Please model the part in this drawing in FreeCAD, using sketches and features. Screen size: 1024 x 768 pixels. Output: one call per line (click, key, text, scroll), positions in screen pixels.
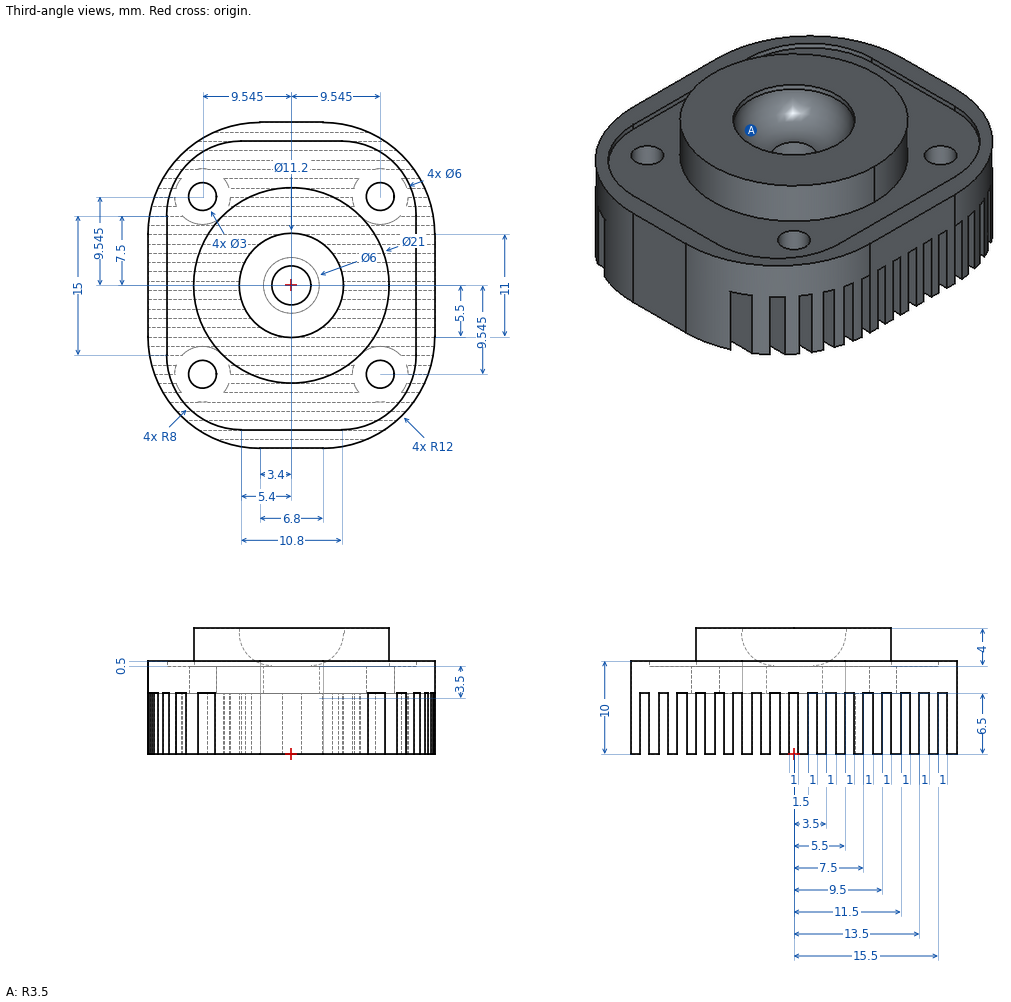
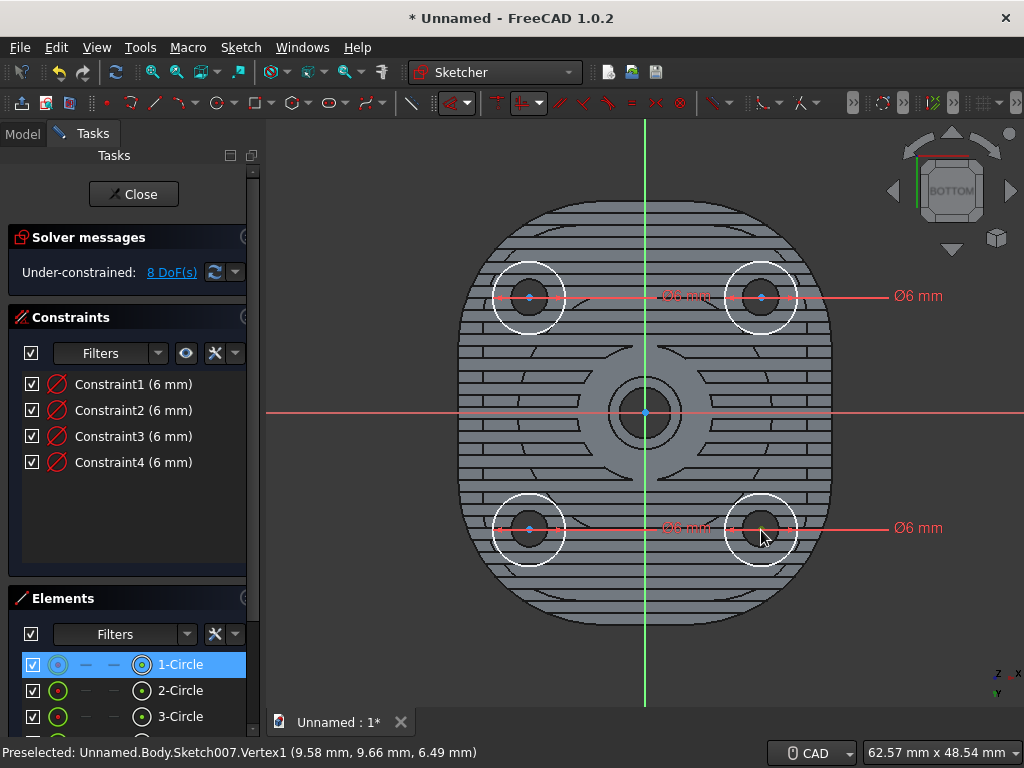
click(529, 530)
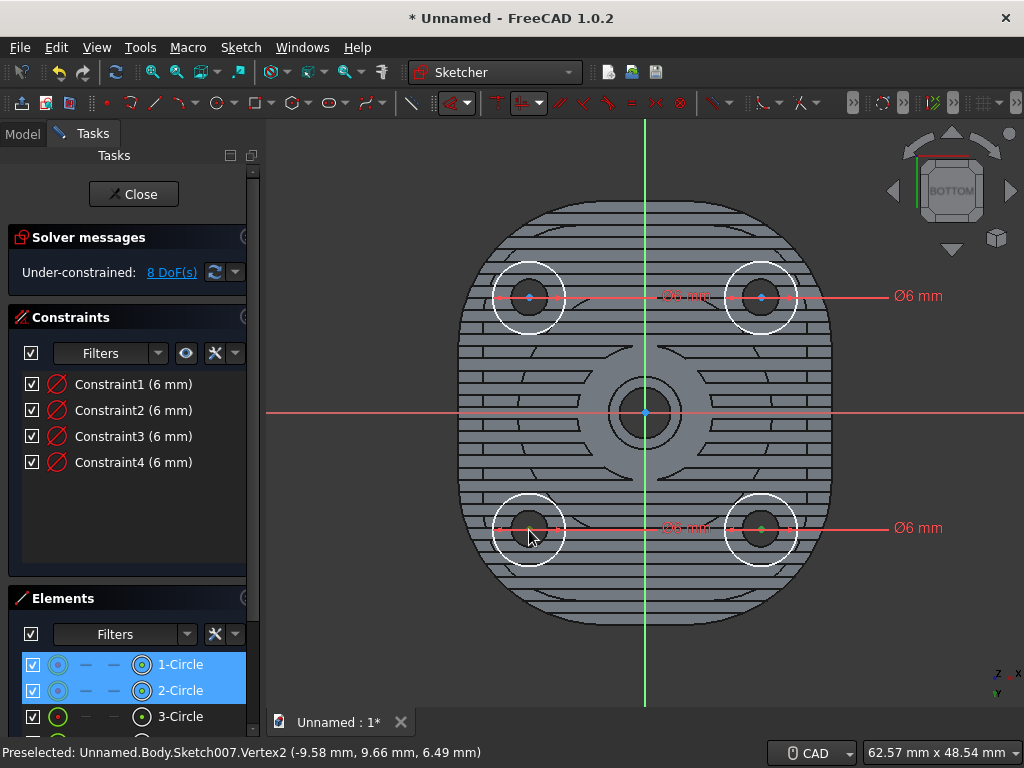
key(h)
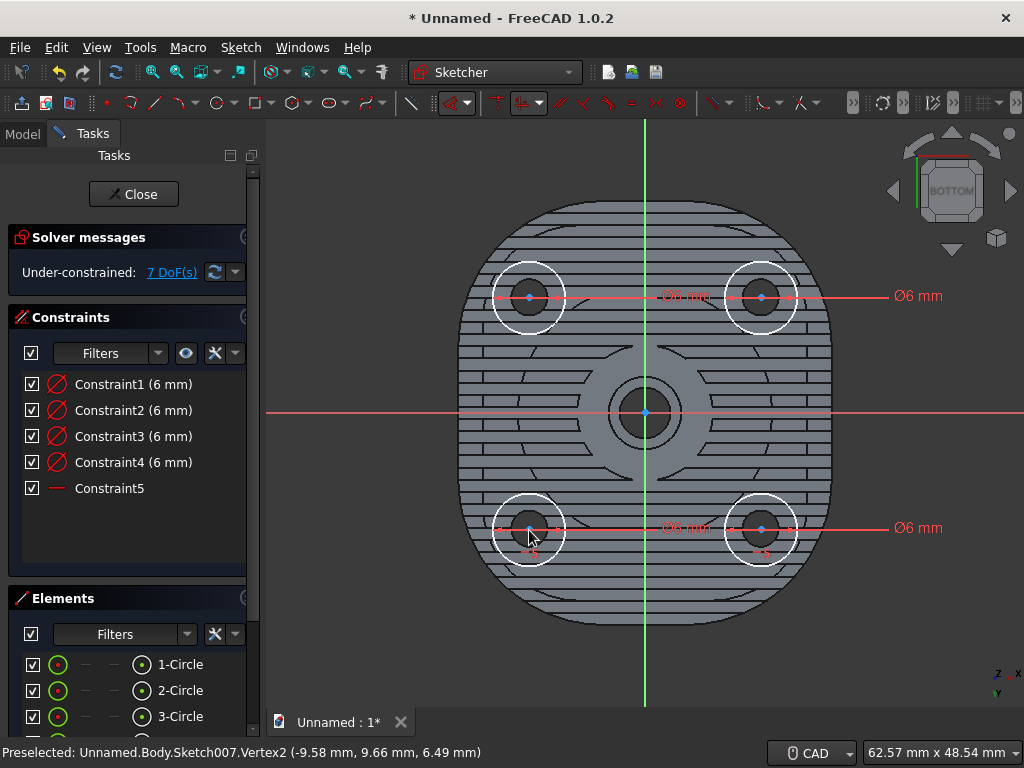
click(761, 530)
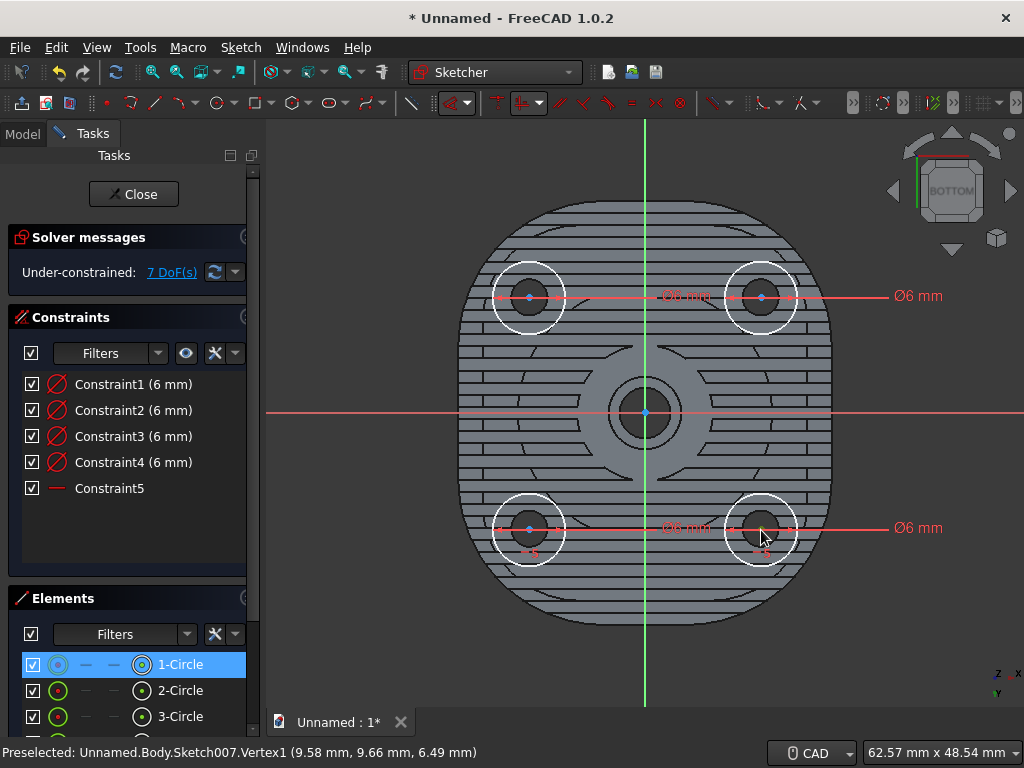
click(761, 298)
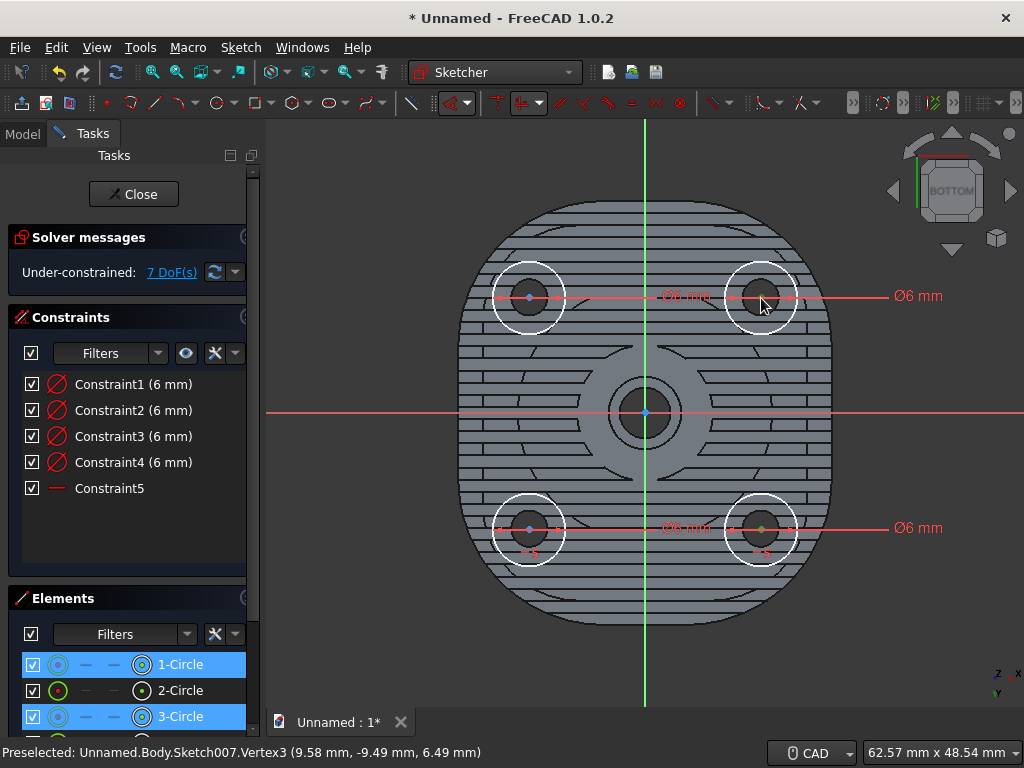
key(v)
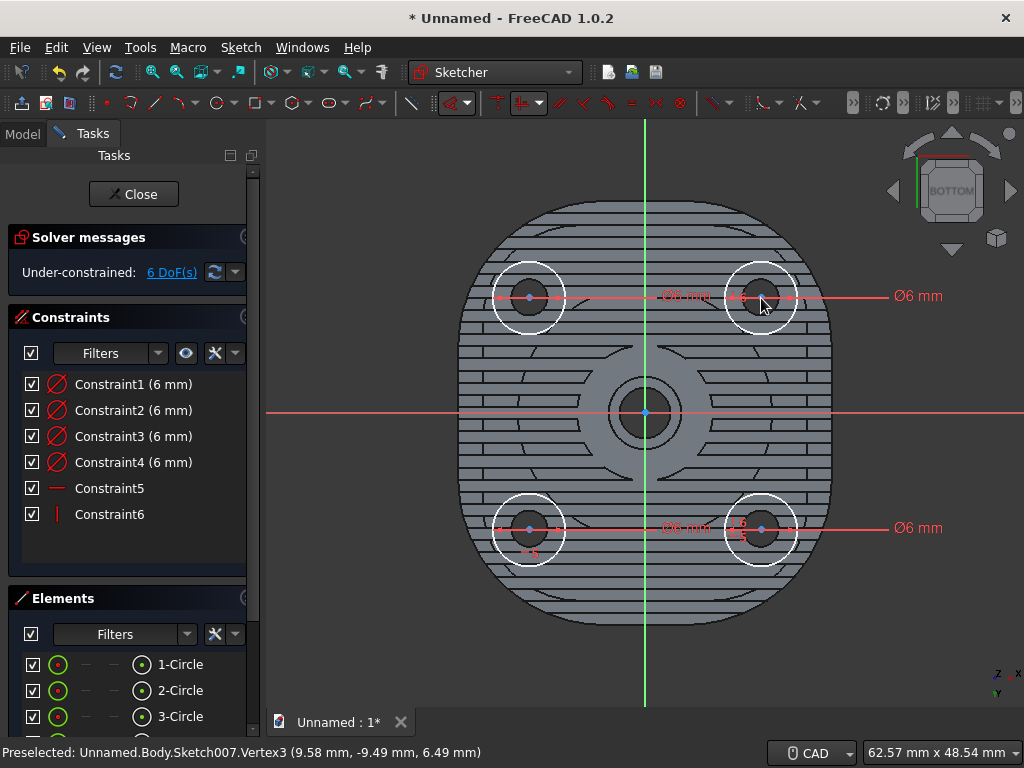
click(529, 530)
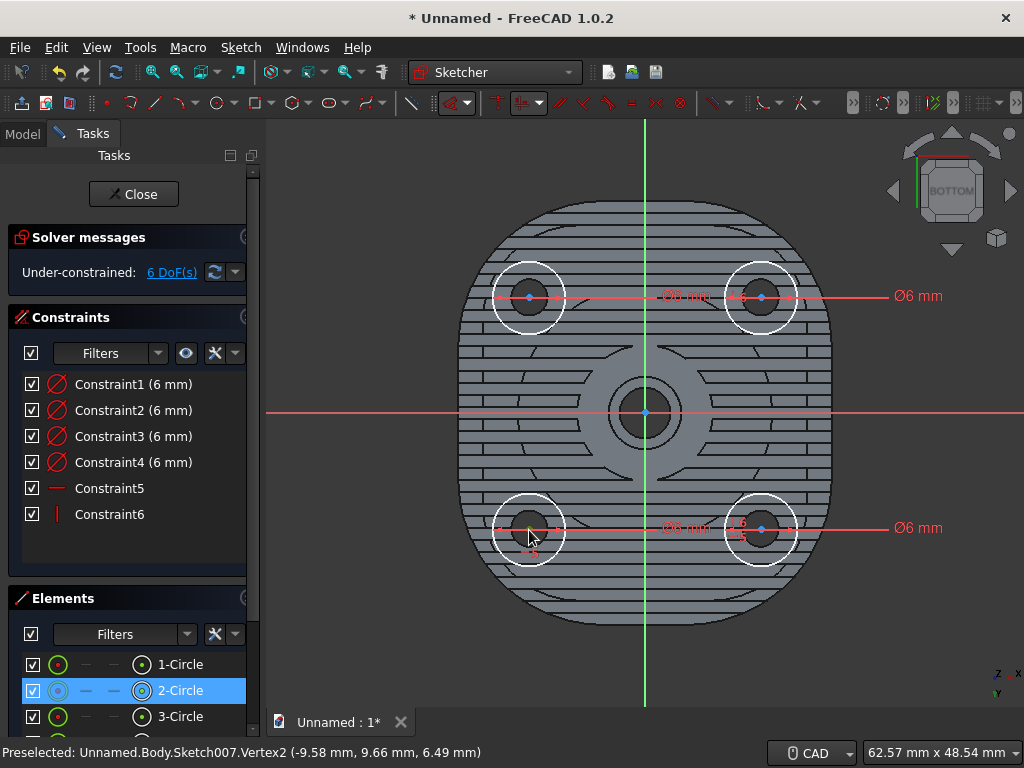
click(529, 298)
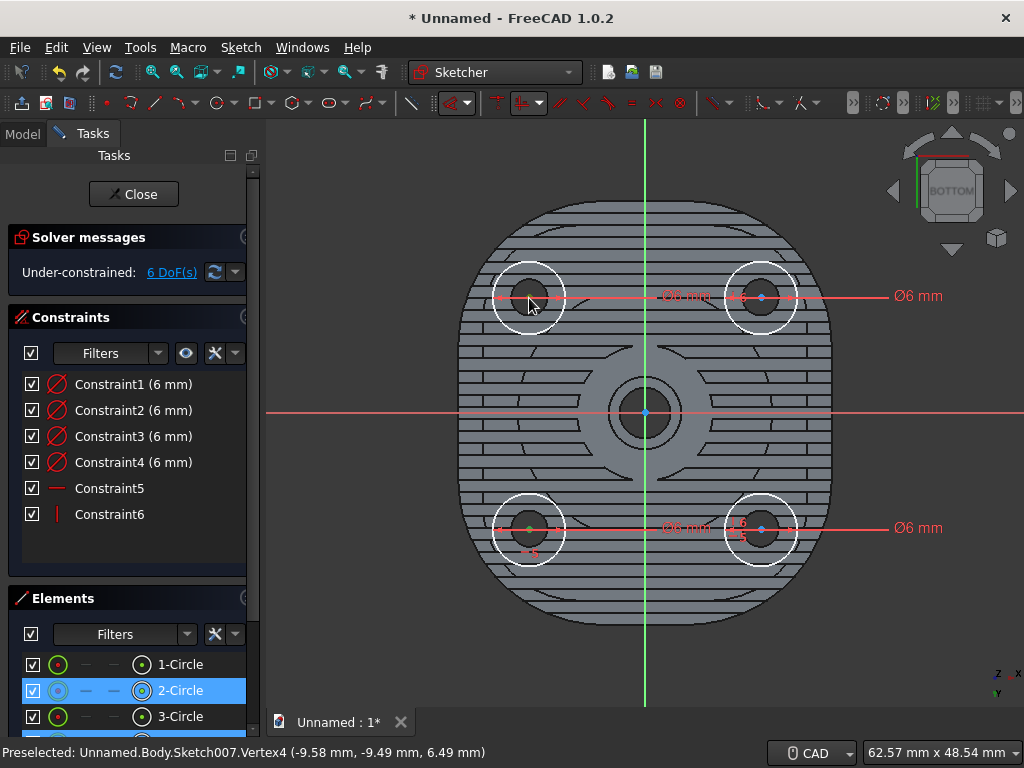
click(542, 104)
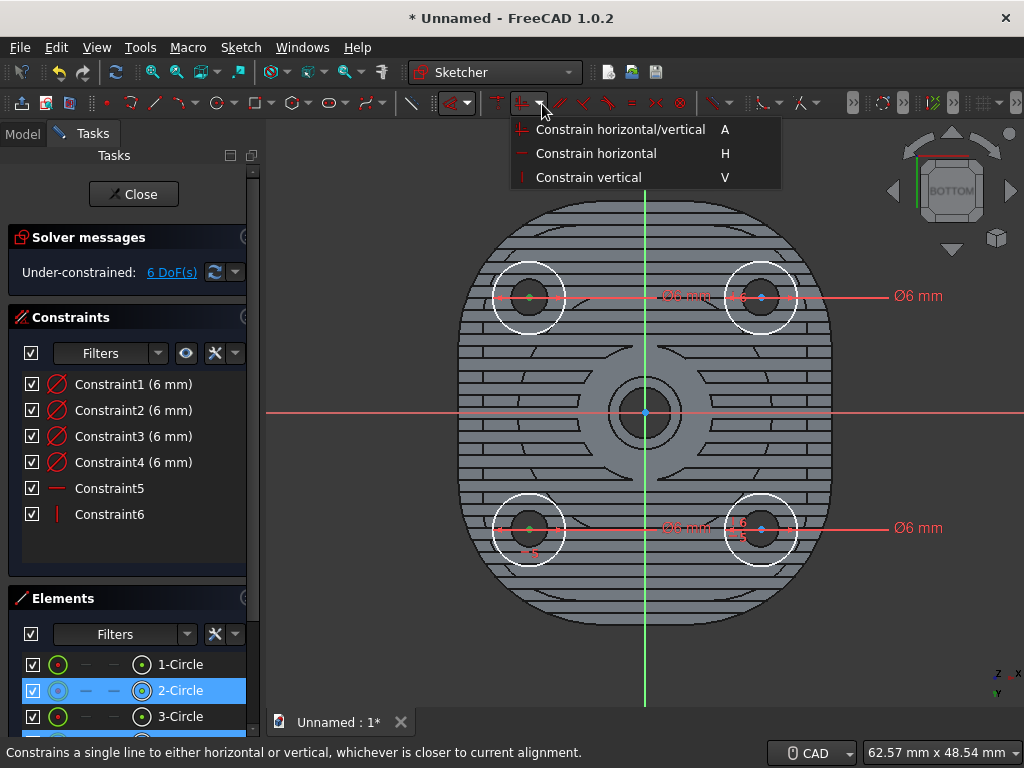
click(646, 177)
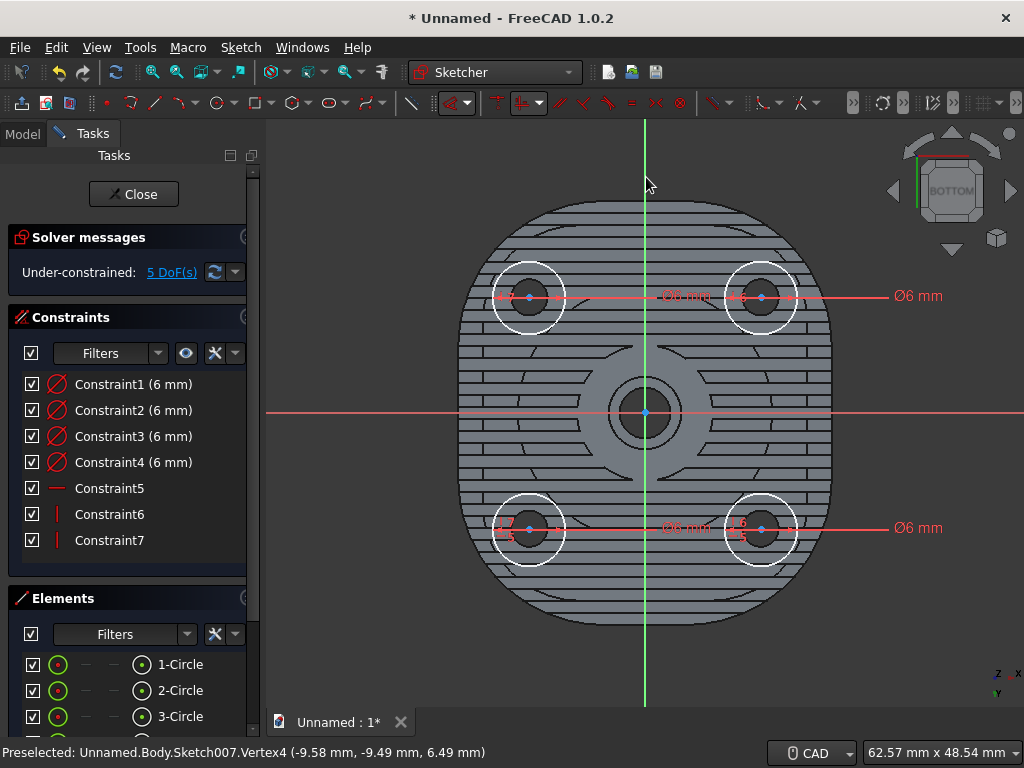
click(761, 298)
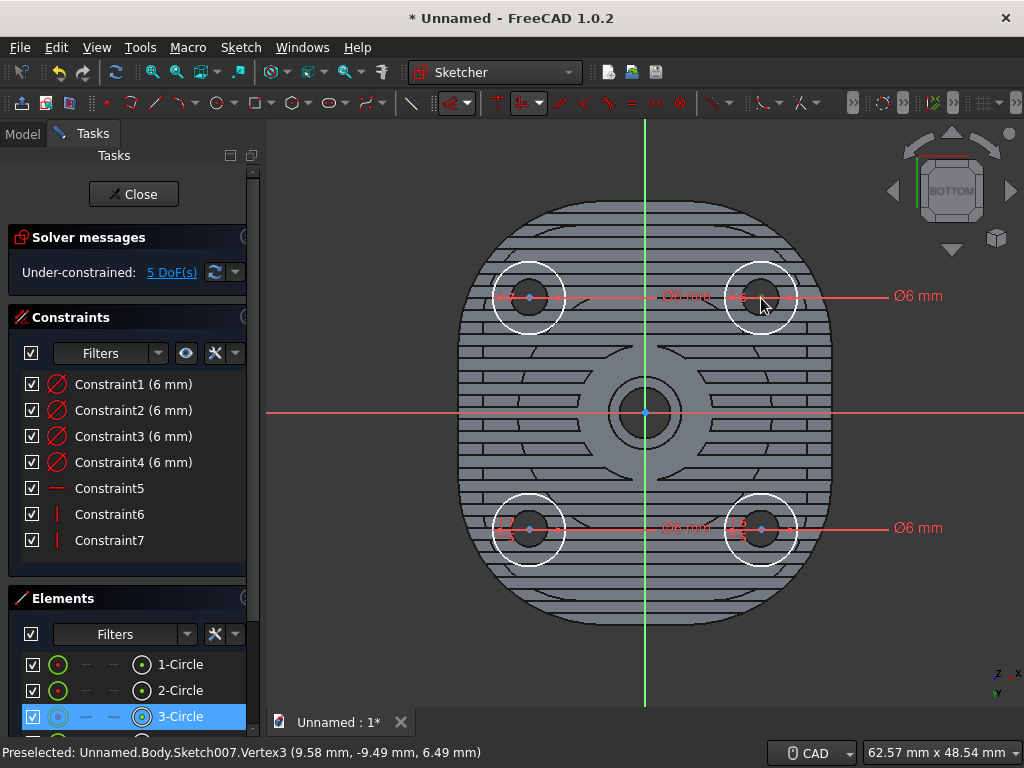
click(529, 298)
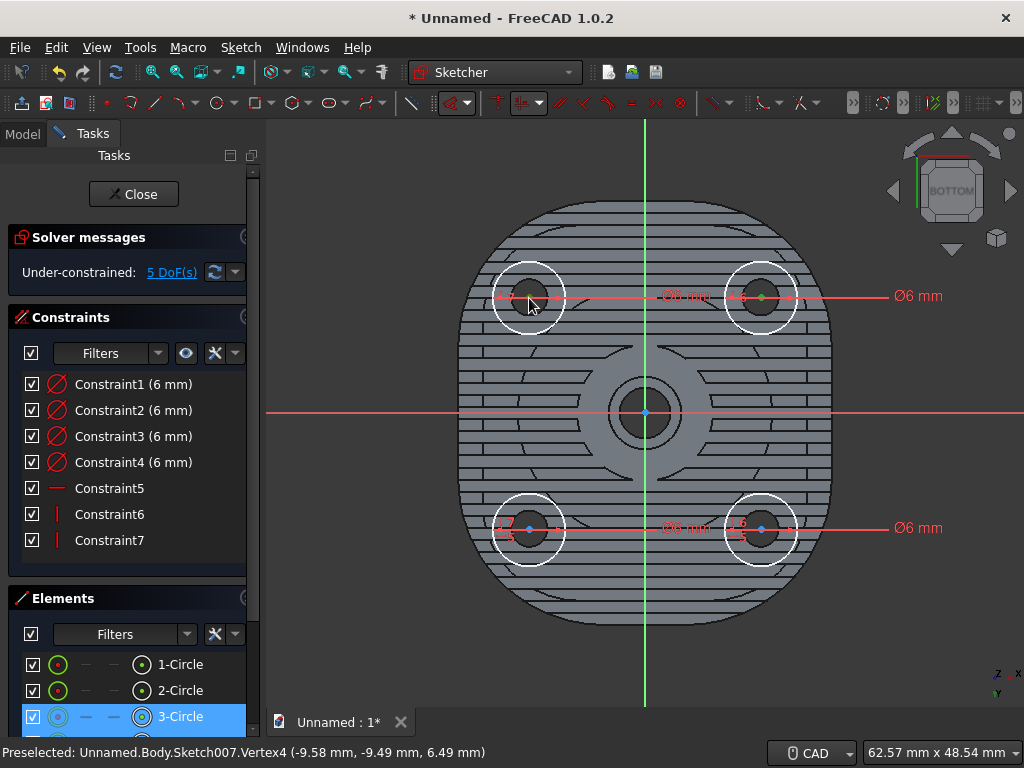
click(542, 104)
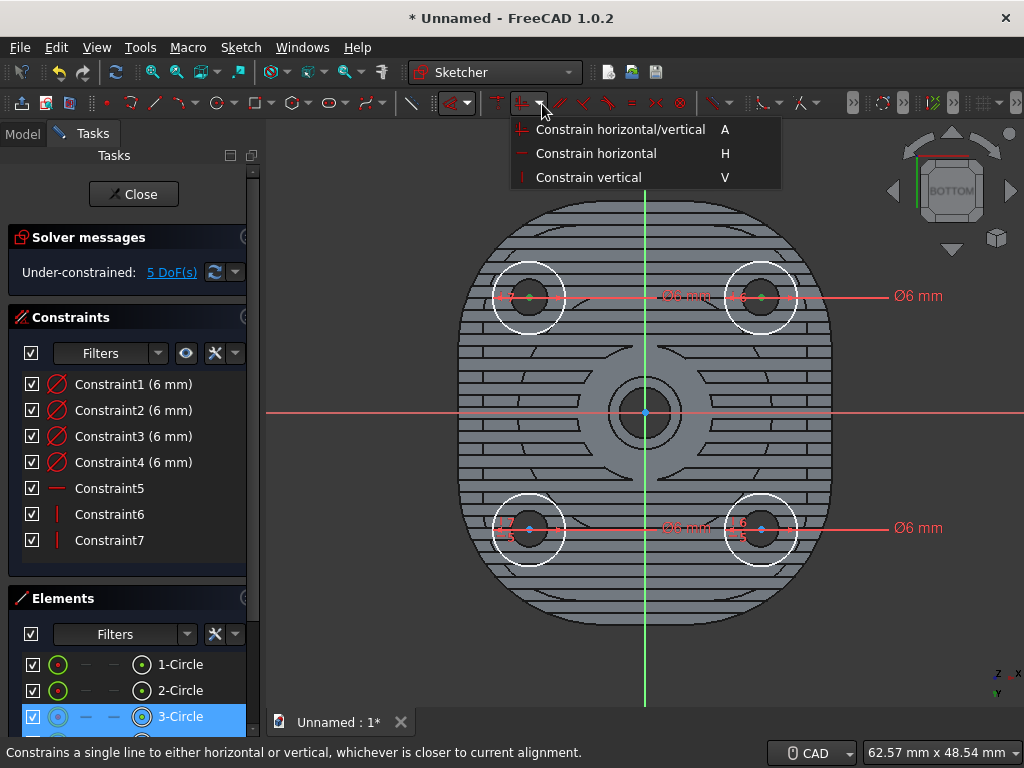
click(646, 153)